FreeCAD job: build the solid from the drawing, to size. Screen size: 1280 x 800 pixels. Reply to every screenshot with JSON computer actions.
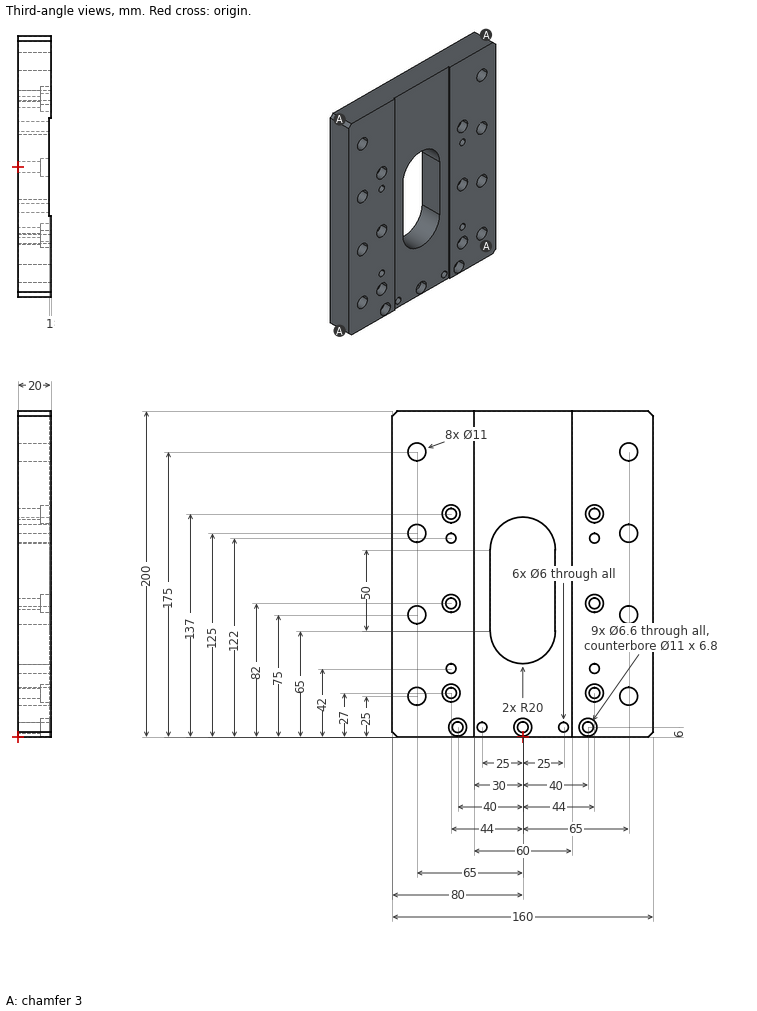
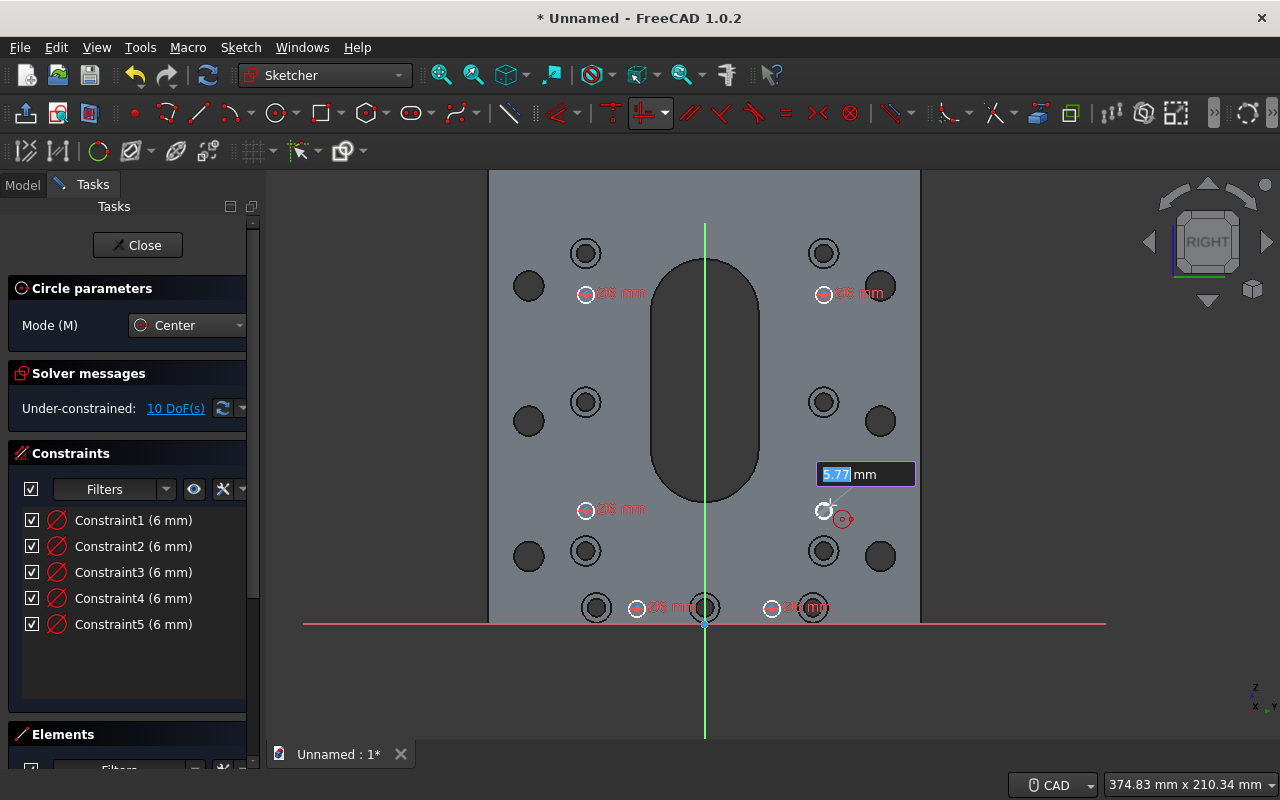
{"action": "type", "text": "6"}
{"action": "key", "text": "Return"}
{"action": "key", "text": "Escape"}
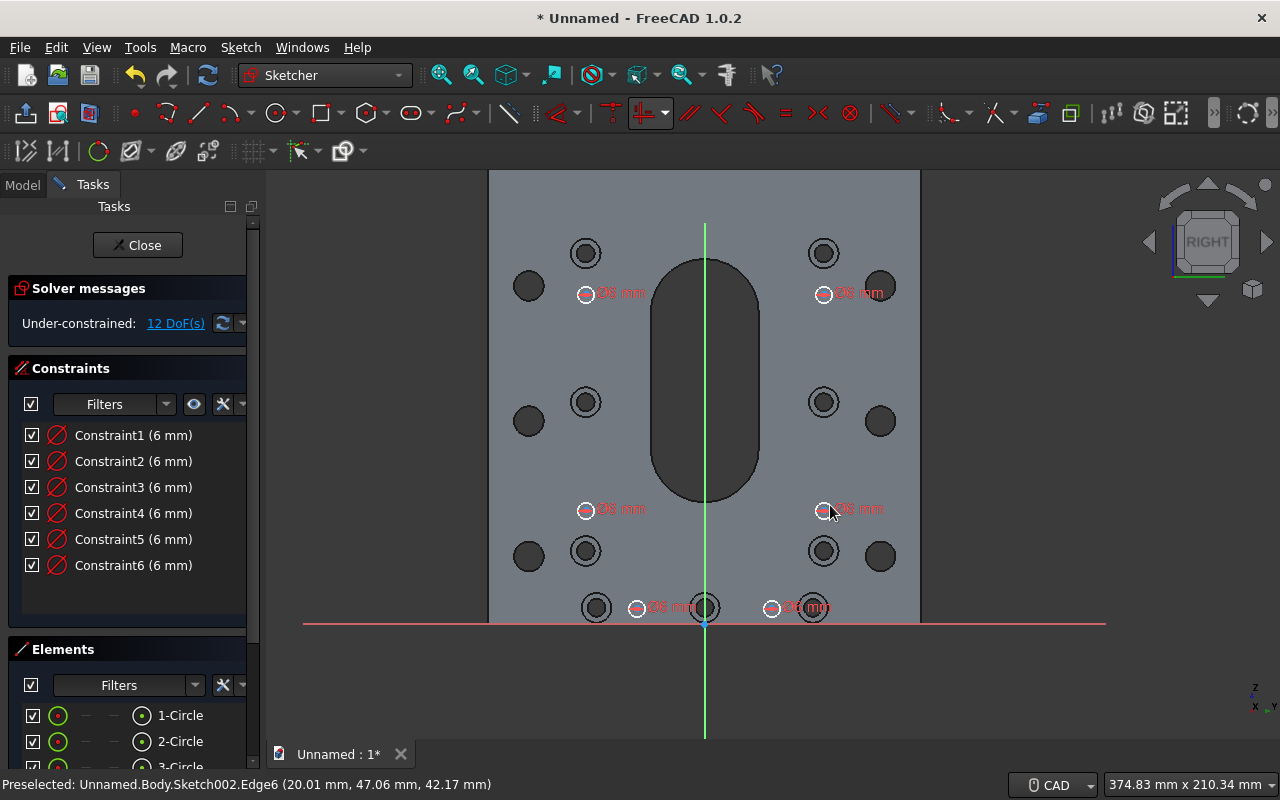
{"action": "left_click", "coordinate": [772, 609]}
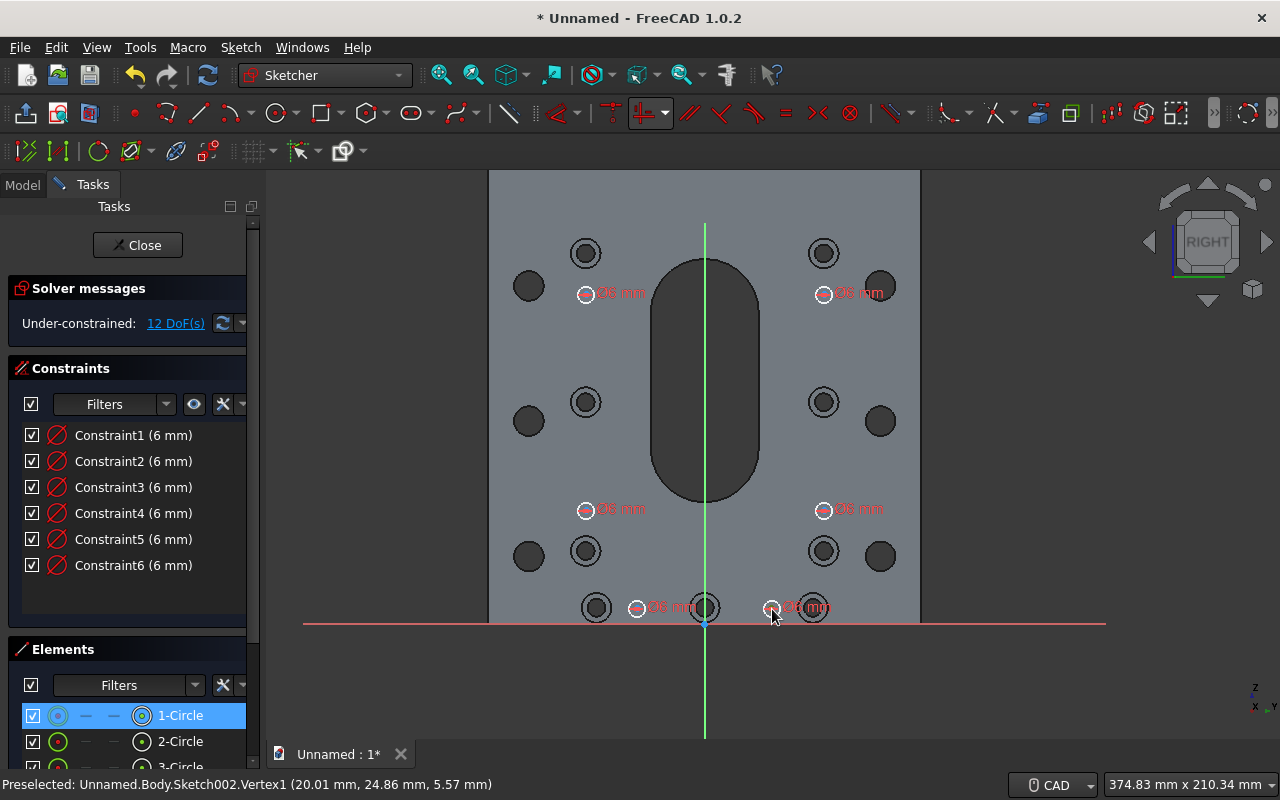
{"action": "left_click", "coordinate": [637, 609]}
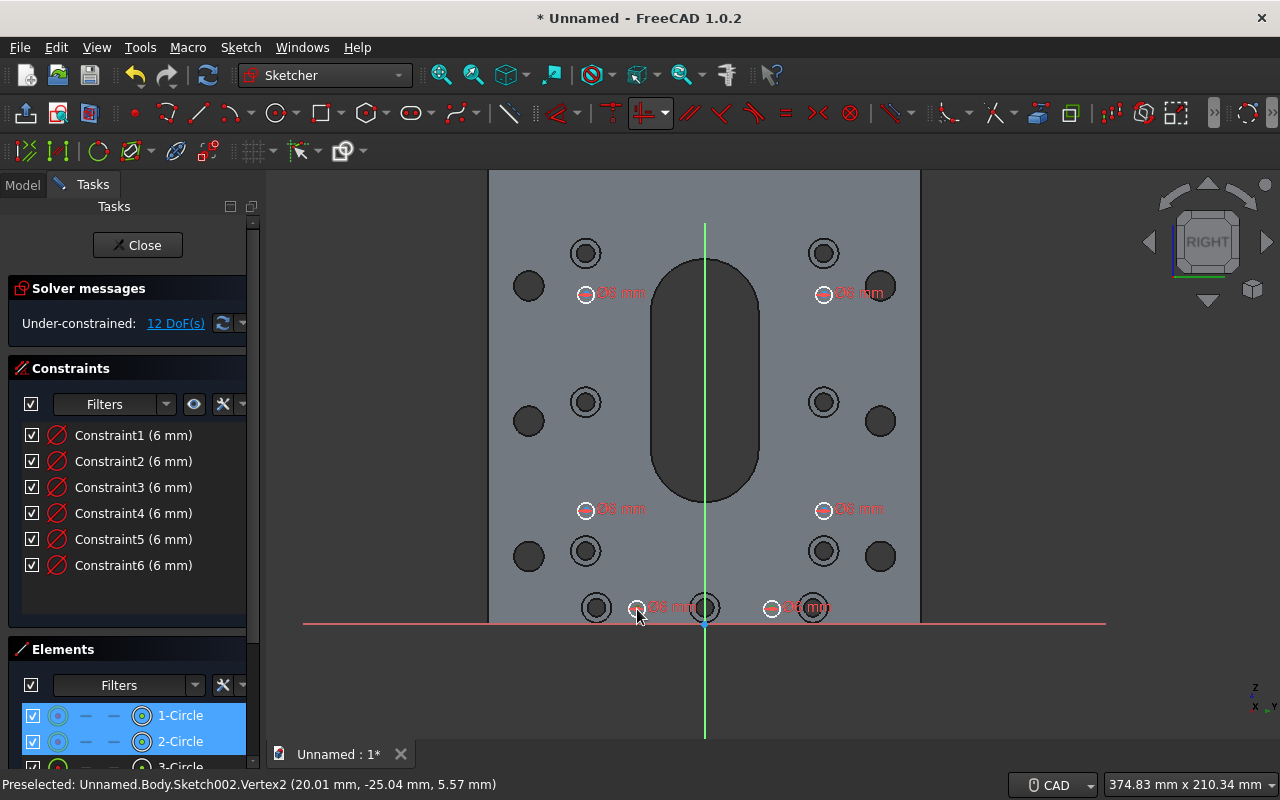
{"action": "key", "text": "h"}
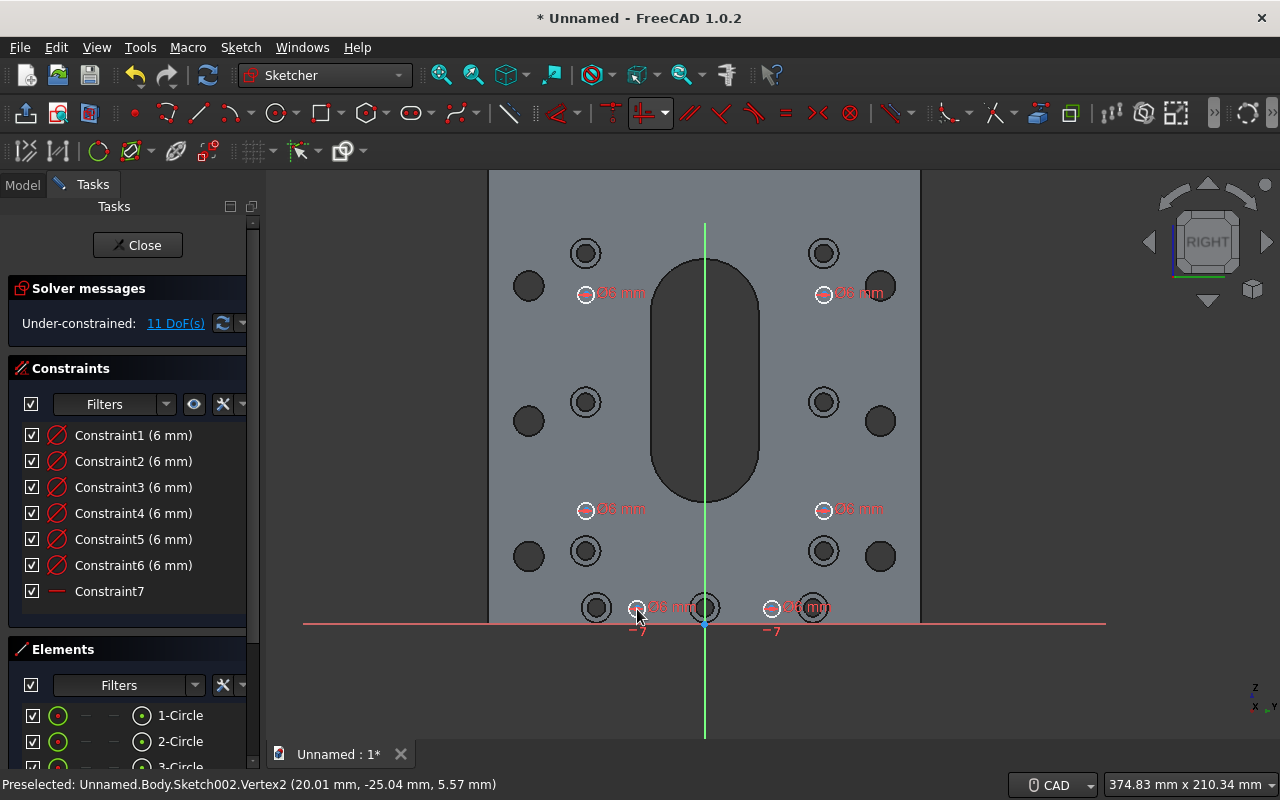
{"action": "left_click", "coordinate": [586, 511]}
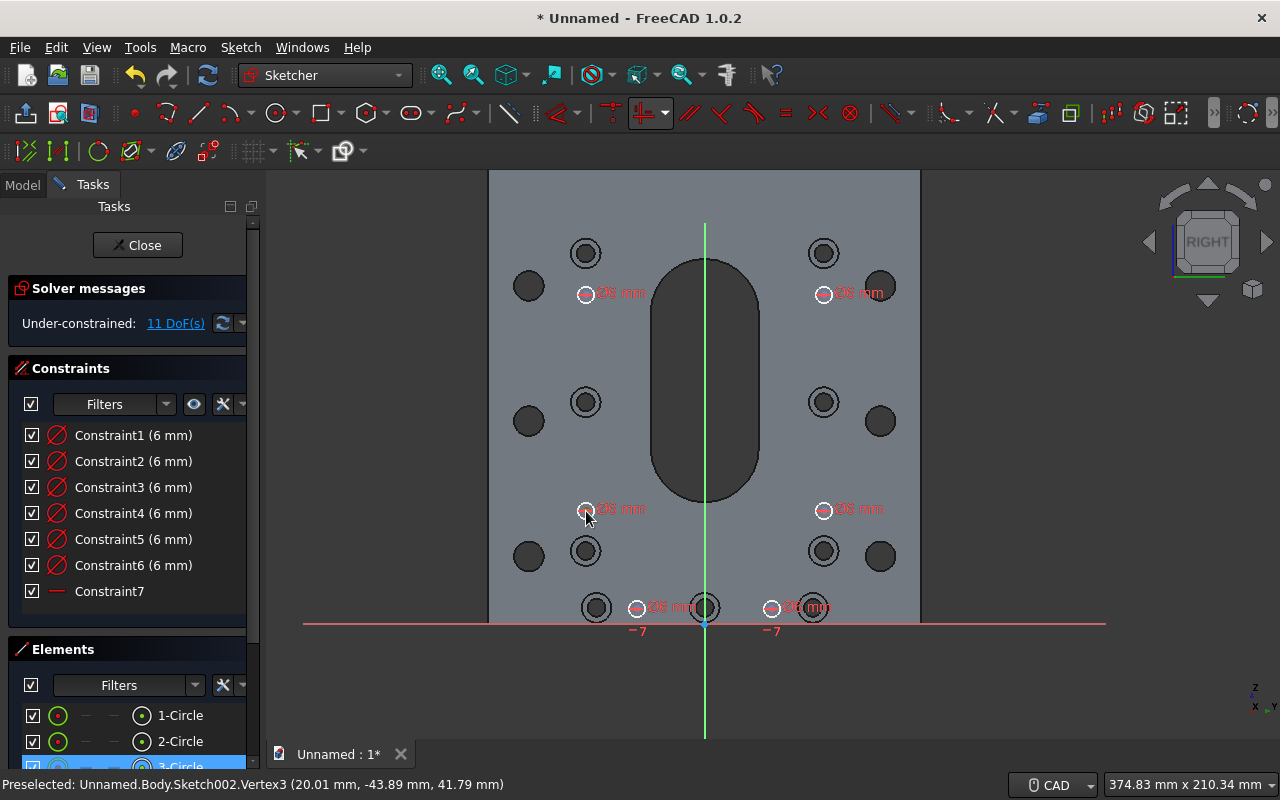
{"action": "left_click", "coordinate": [586, 295]}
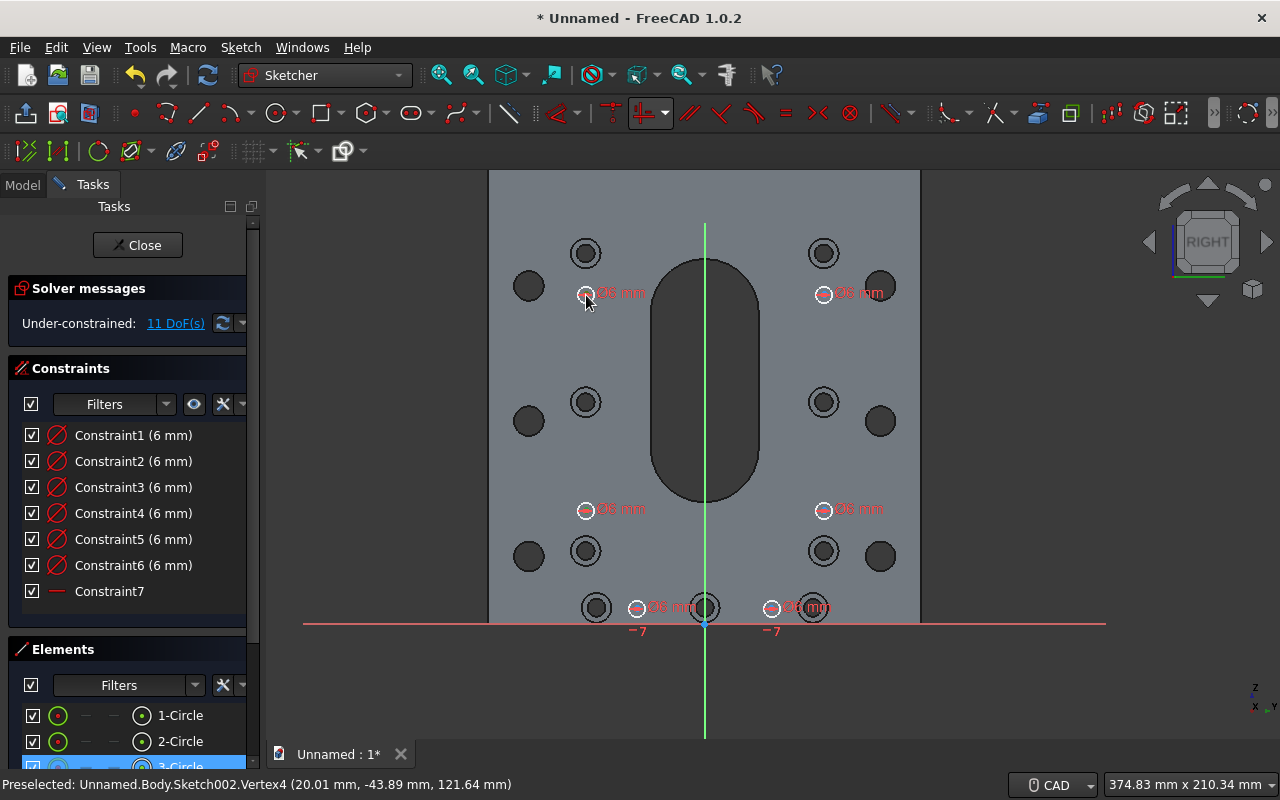
{"action": "key", "text": "v"}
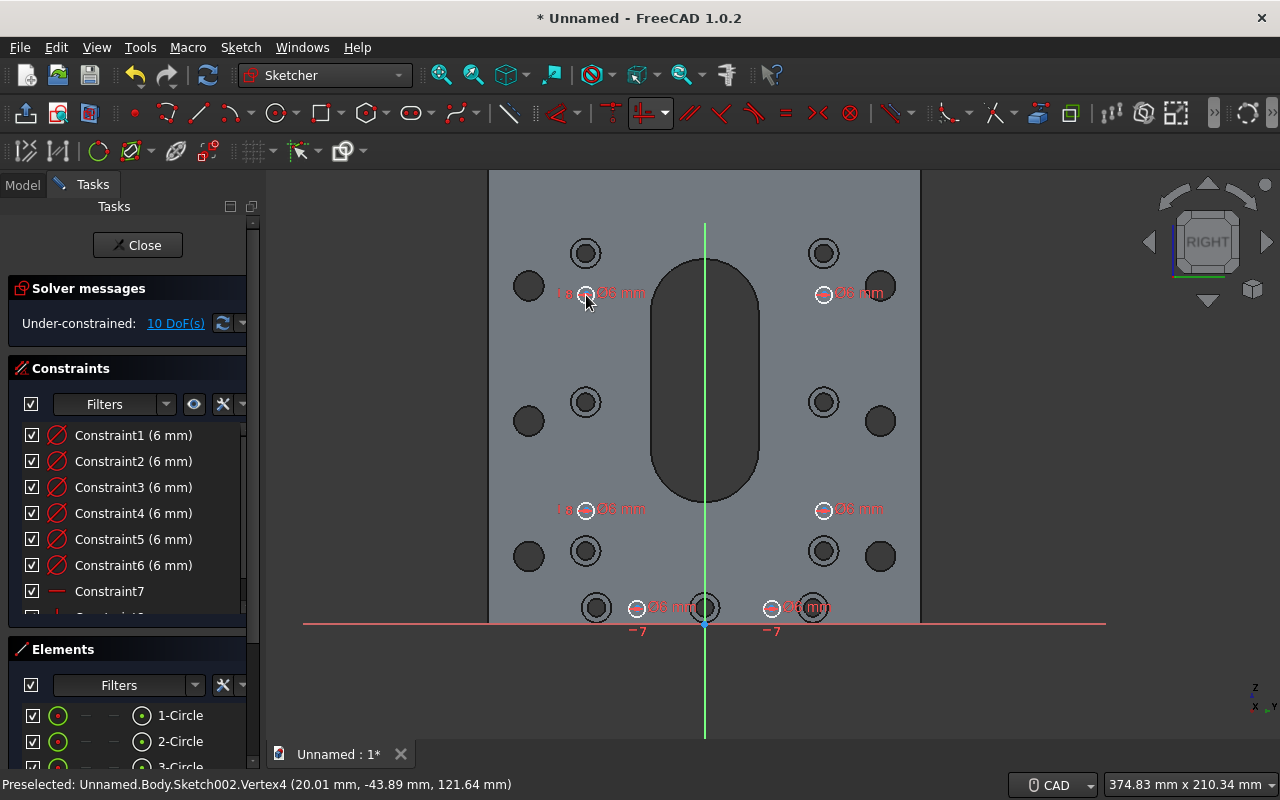
{"action": "left_click", "coordinate": [586, 295]}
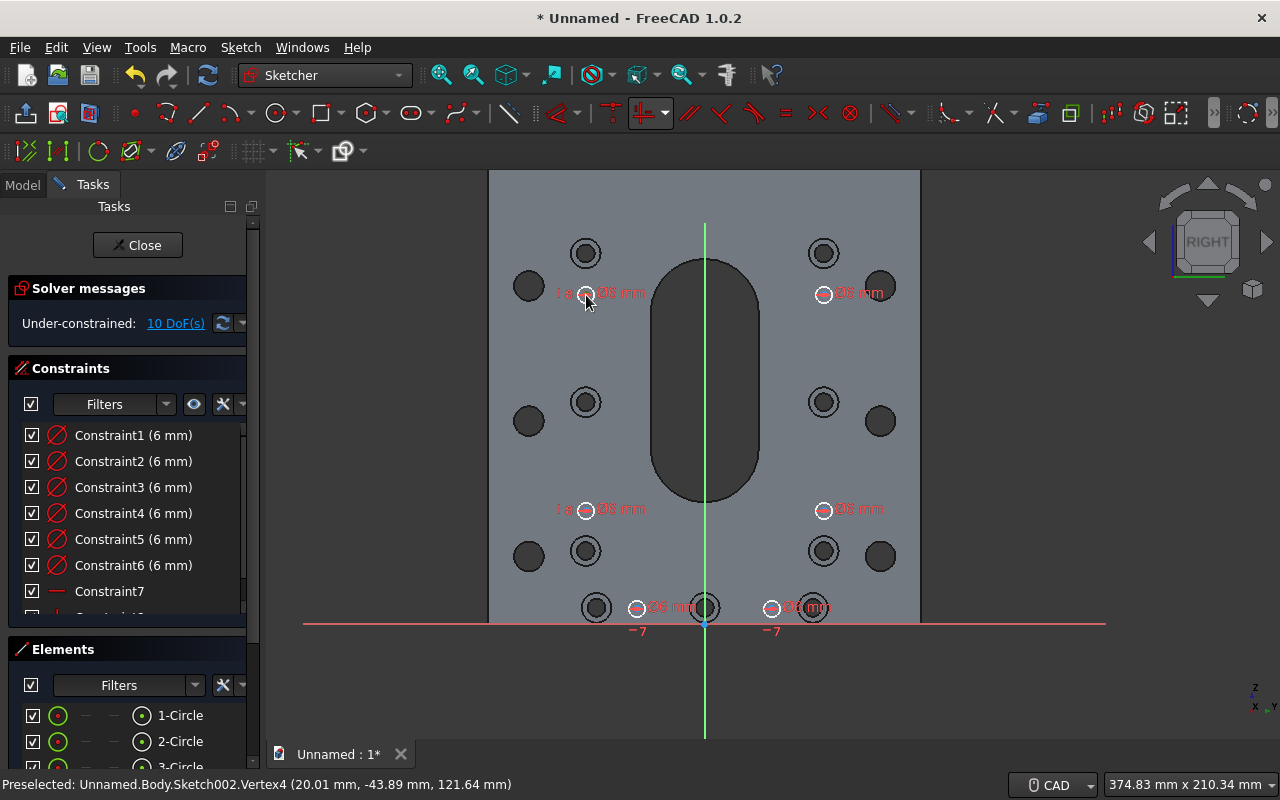
{"action": "left_click", "coordinate": [824, 295]}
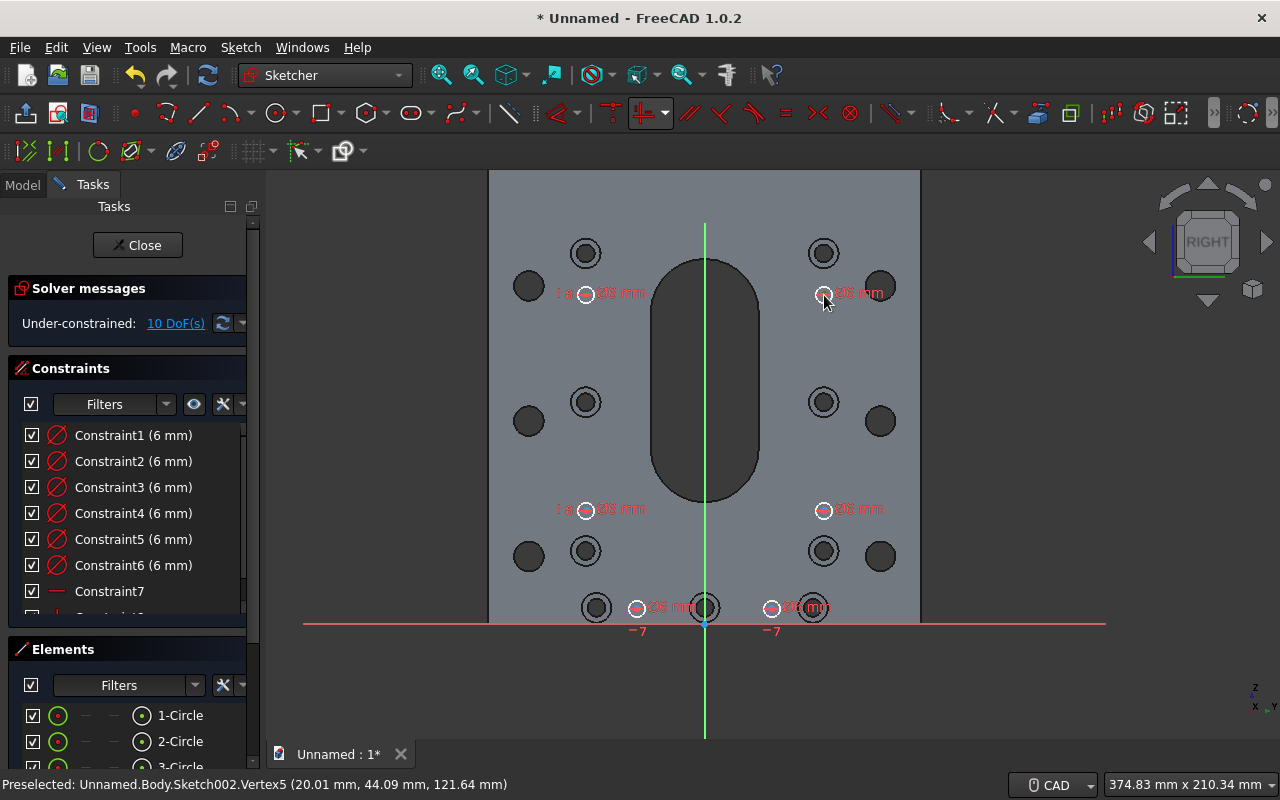
{"action": "key", "text": "h"}